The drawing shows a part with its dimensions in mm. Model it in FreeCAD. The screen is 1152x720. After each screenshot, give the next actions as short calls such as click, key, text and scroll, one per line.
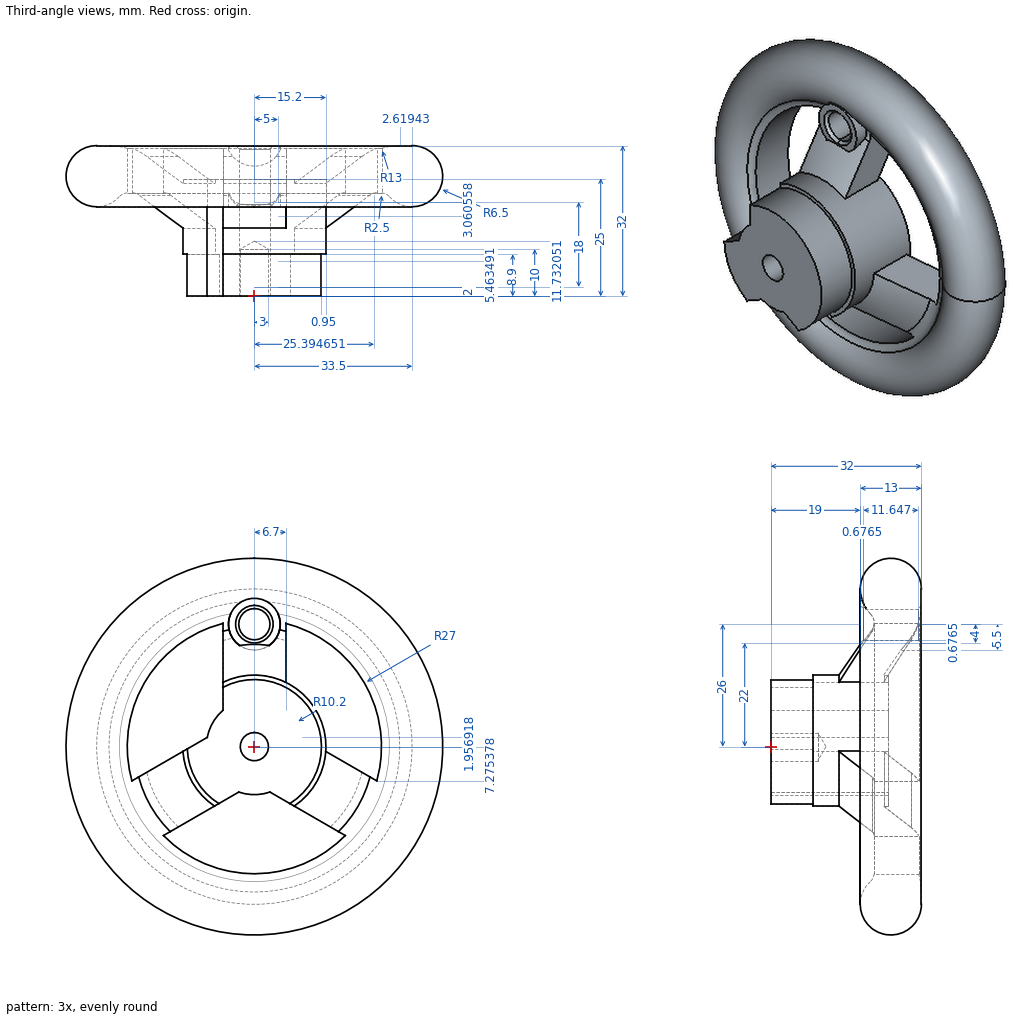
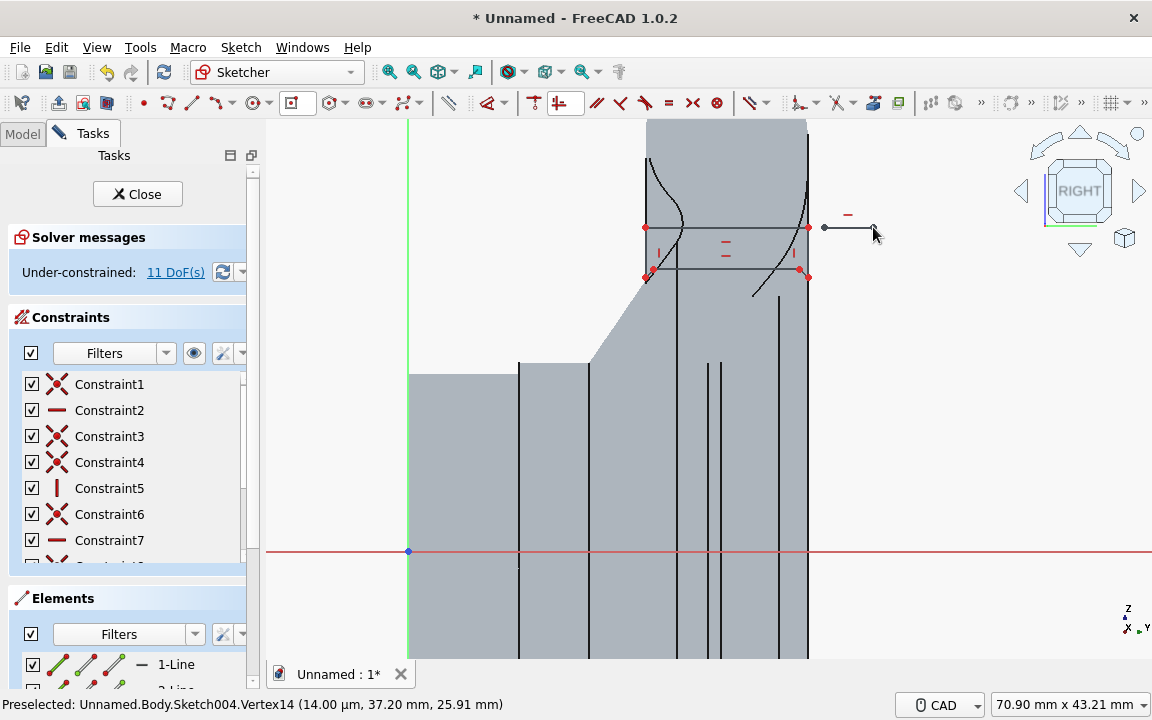
click(839, 228)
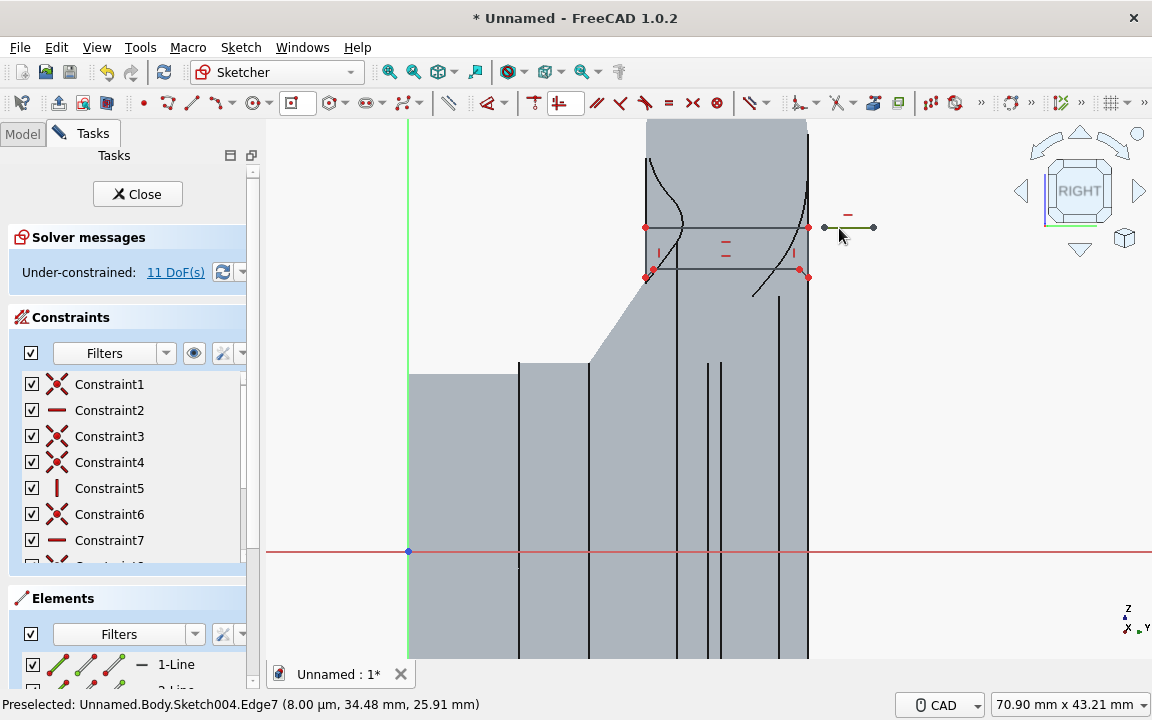
click(450, 104)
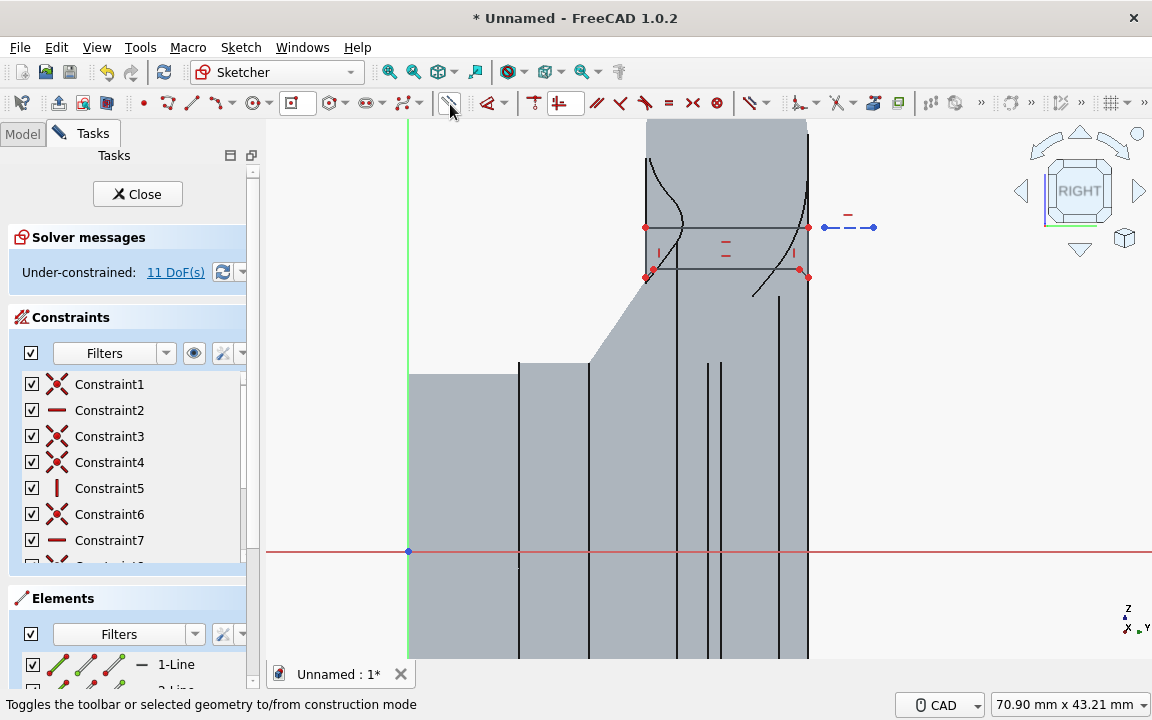
click(488, 104)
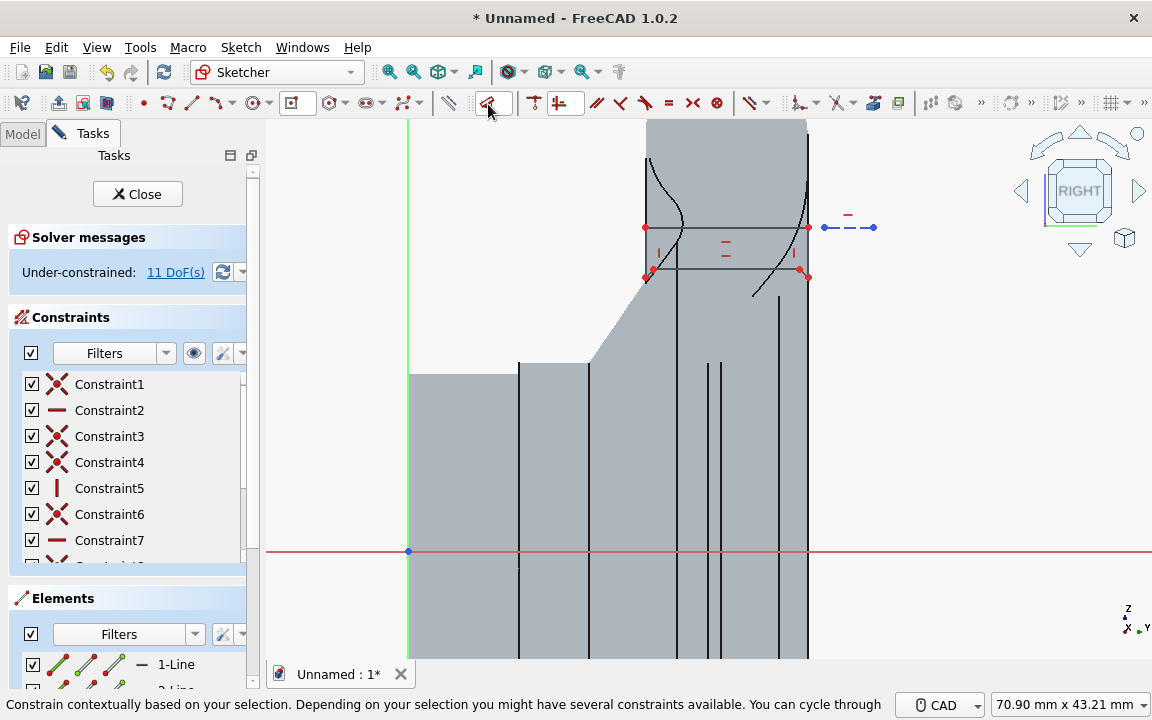
scroll(808, 262, up, 2)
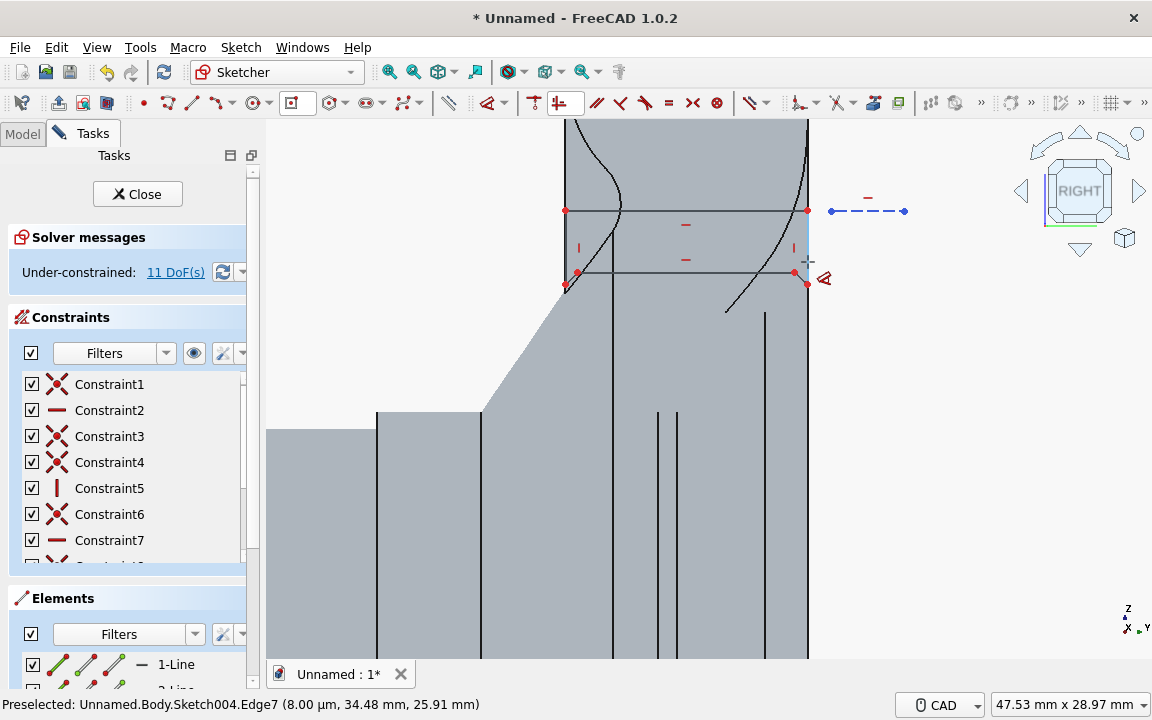
click(808, 262)
click(842, 248)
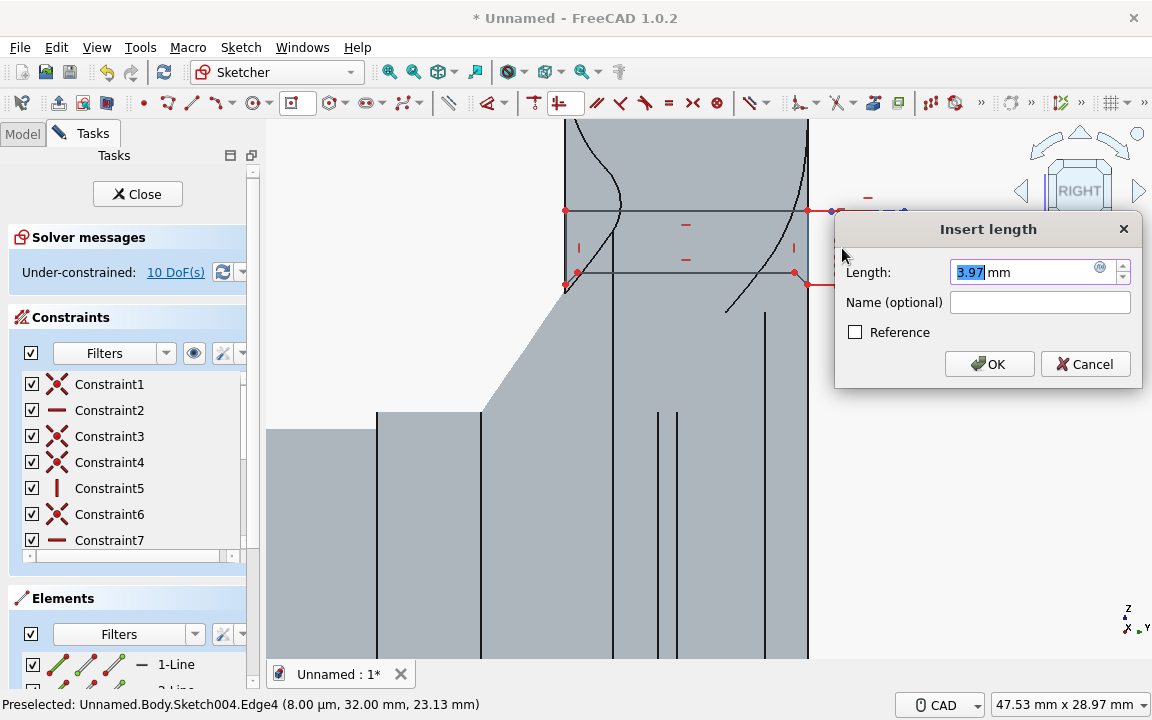
text(4)
key(Return)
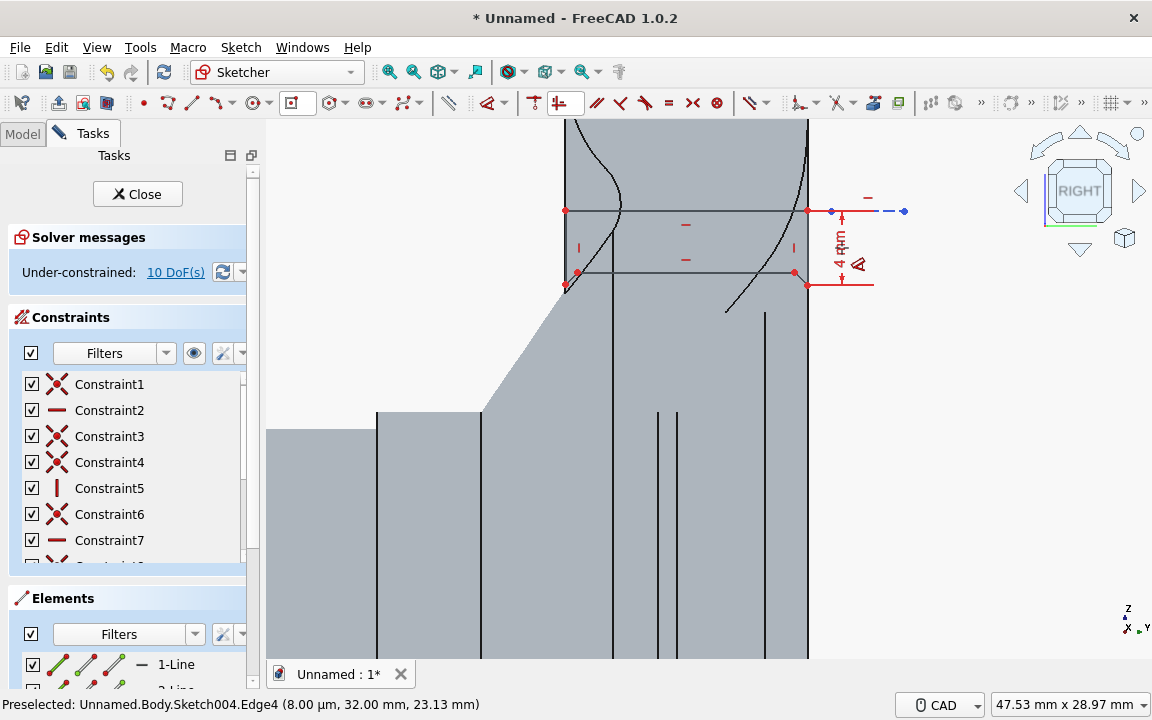
click(566, 233)
click(600, 248)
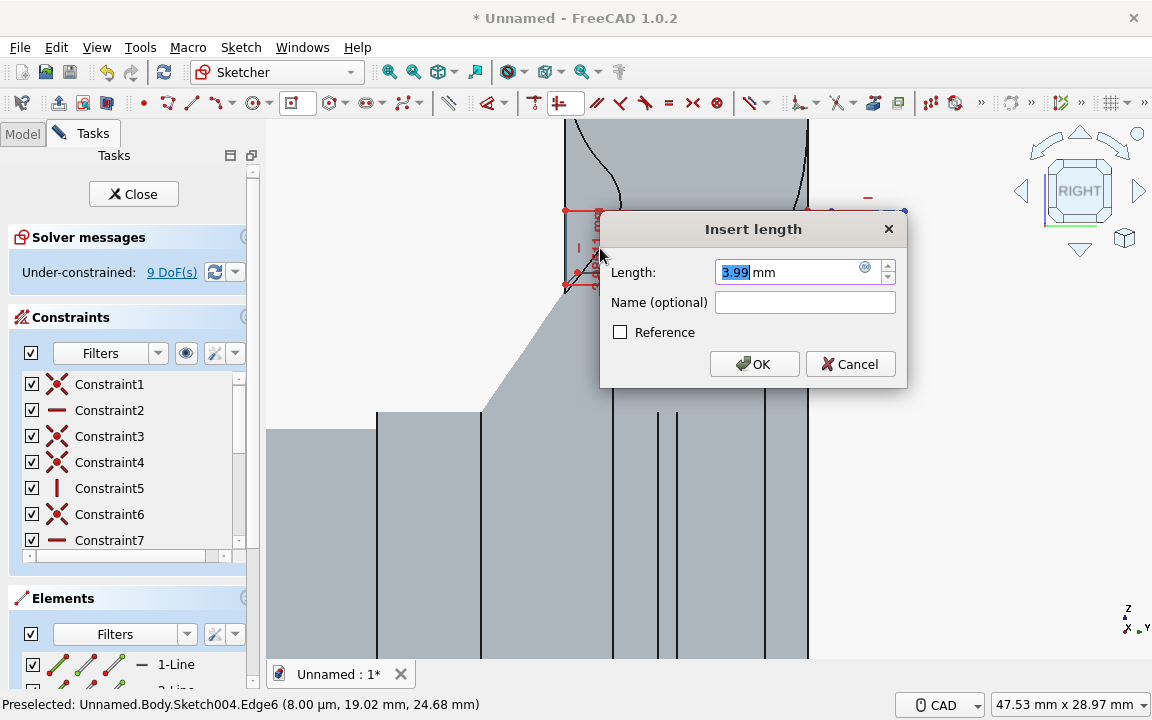
text(4)
key(Return)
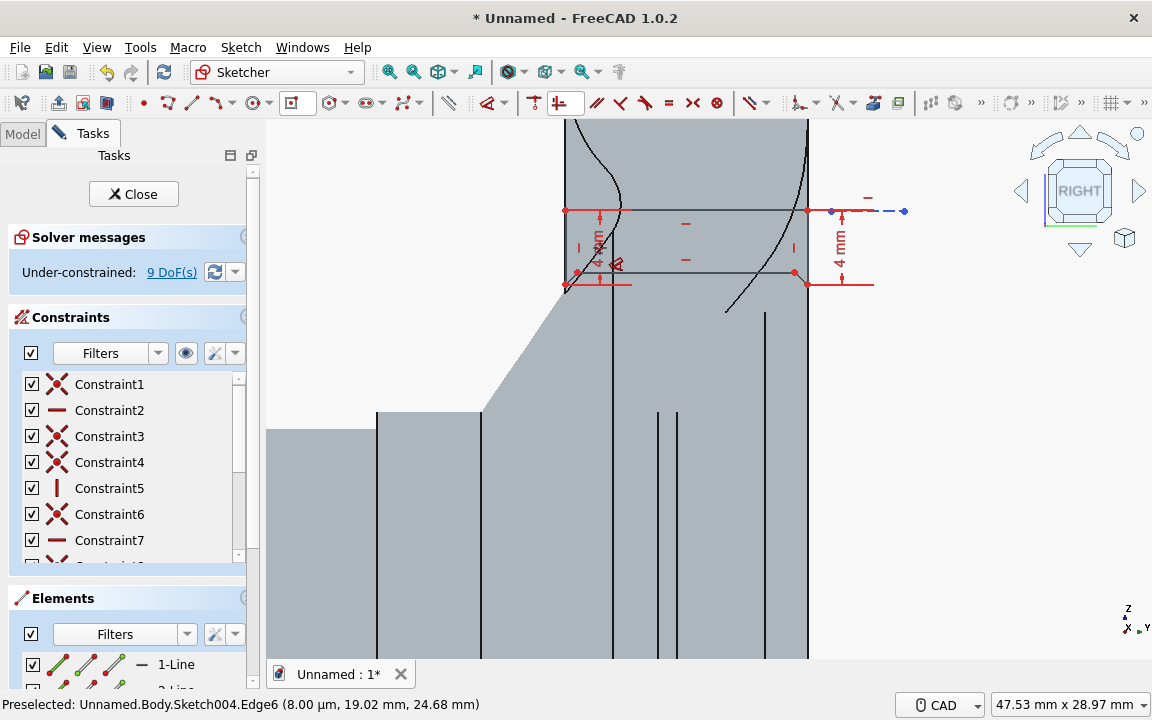
click(735, 210)
click(687, 176)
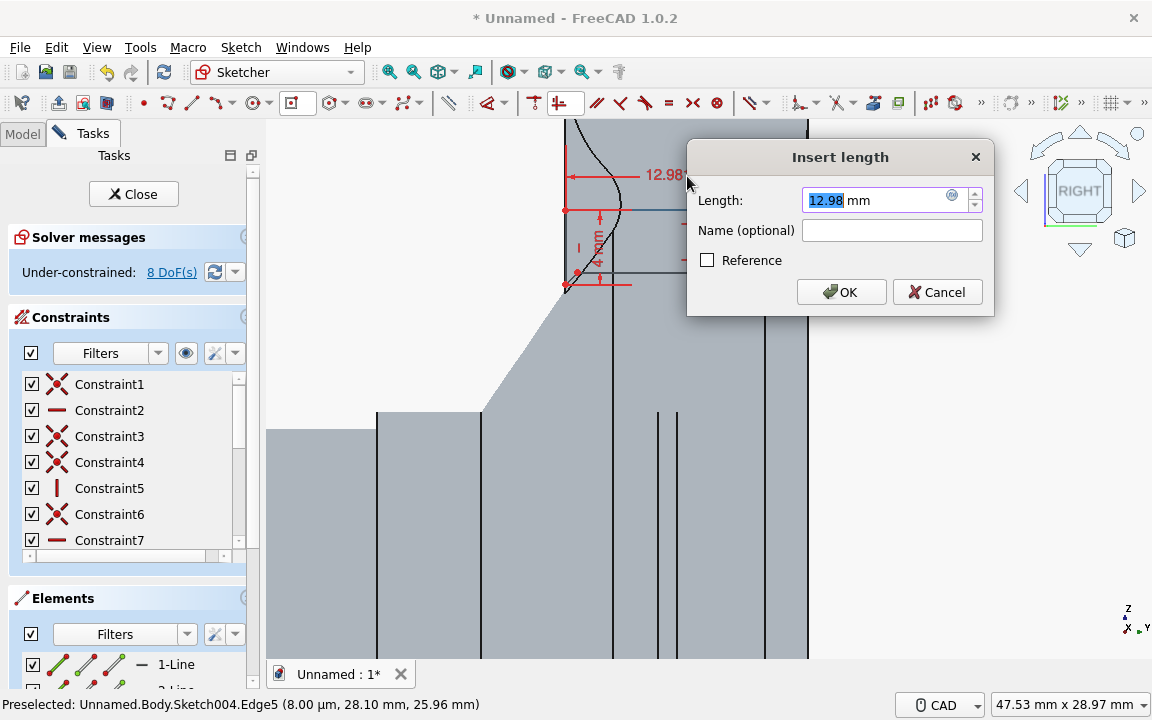
text(13)
key(Return)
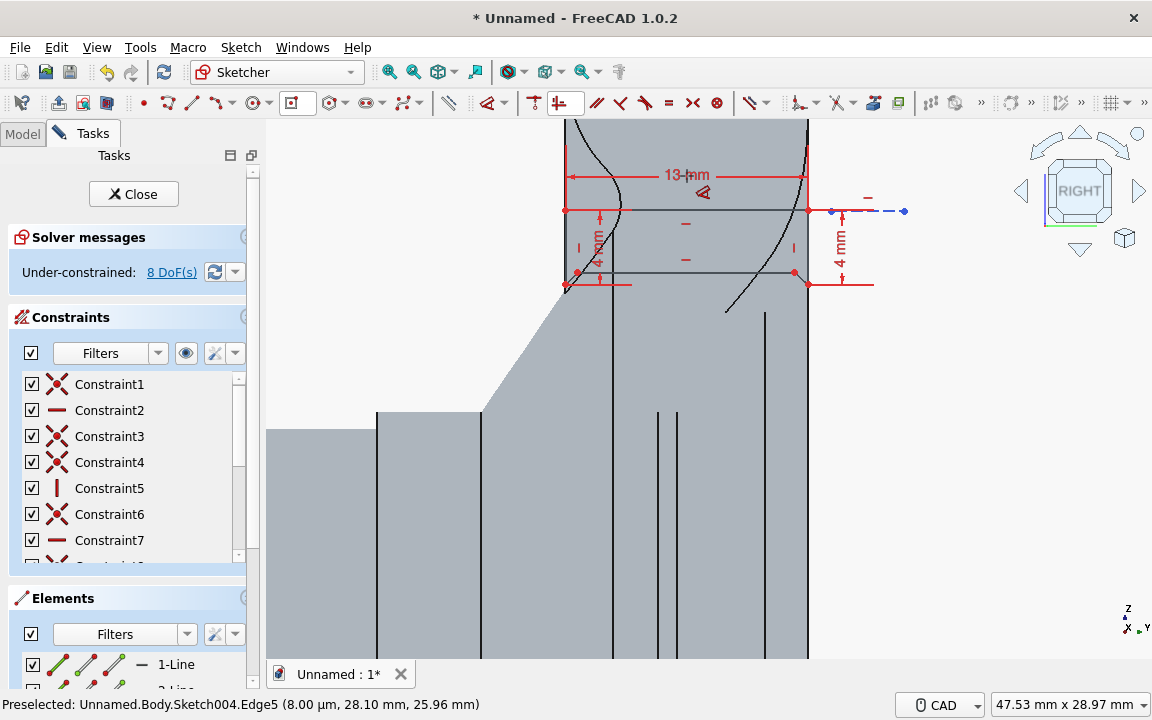
click(566, 285)
click(430, 251)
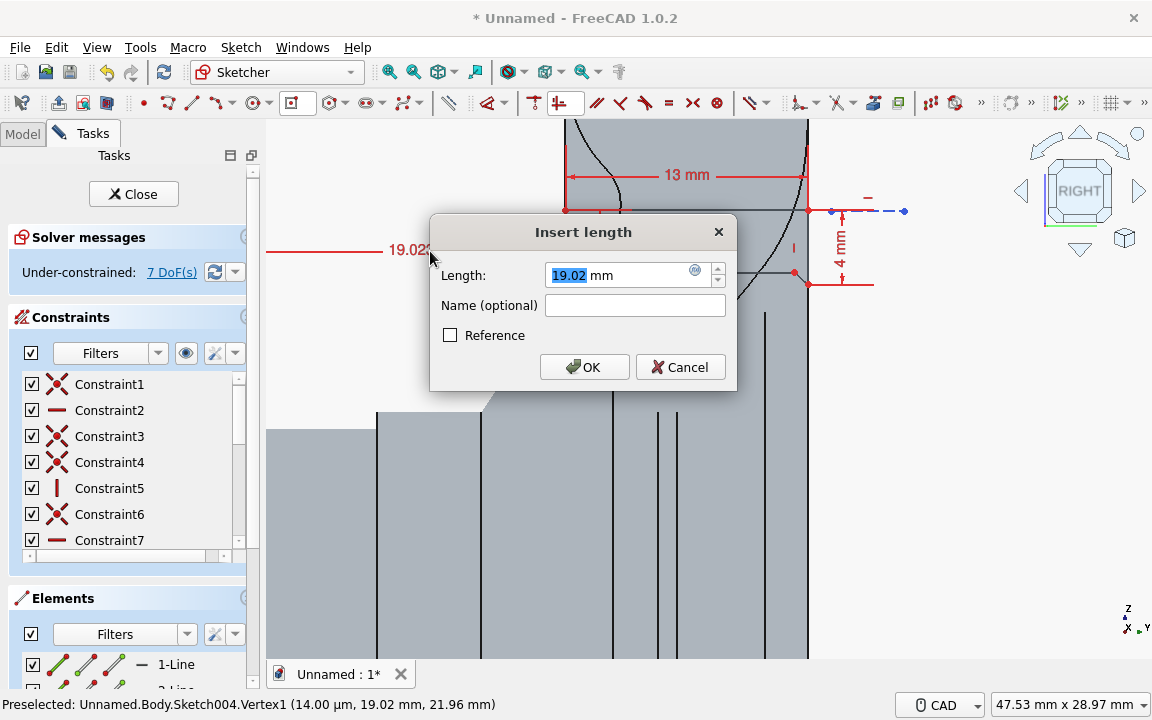
text(19)
key(Return)